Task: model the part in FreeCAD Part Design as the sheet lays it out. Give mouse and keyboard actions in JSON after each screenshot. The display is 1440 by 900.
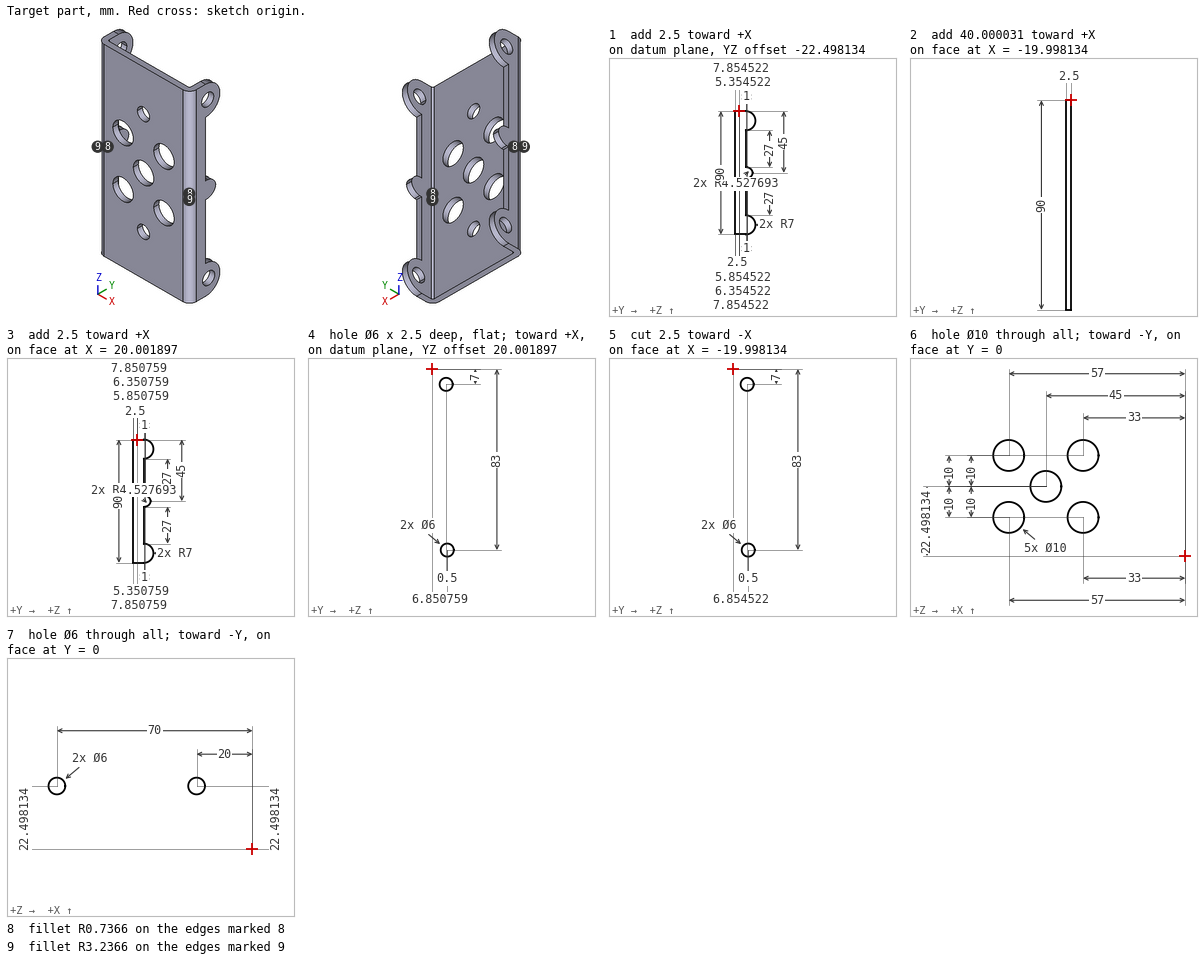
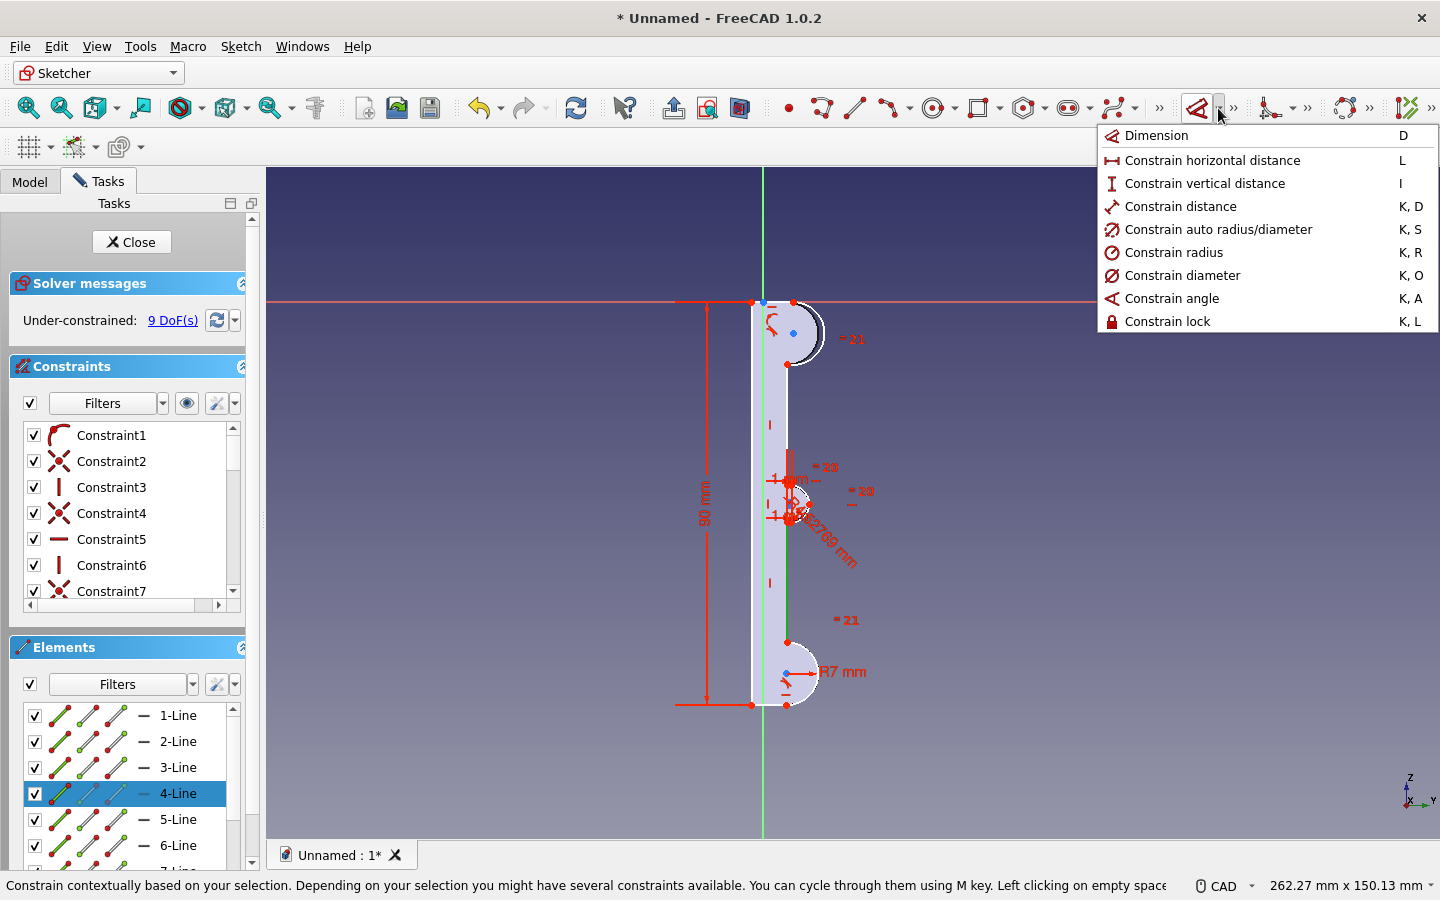
{"action": "left_click", "coordinate": [1268, 184]}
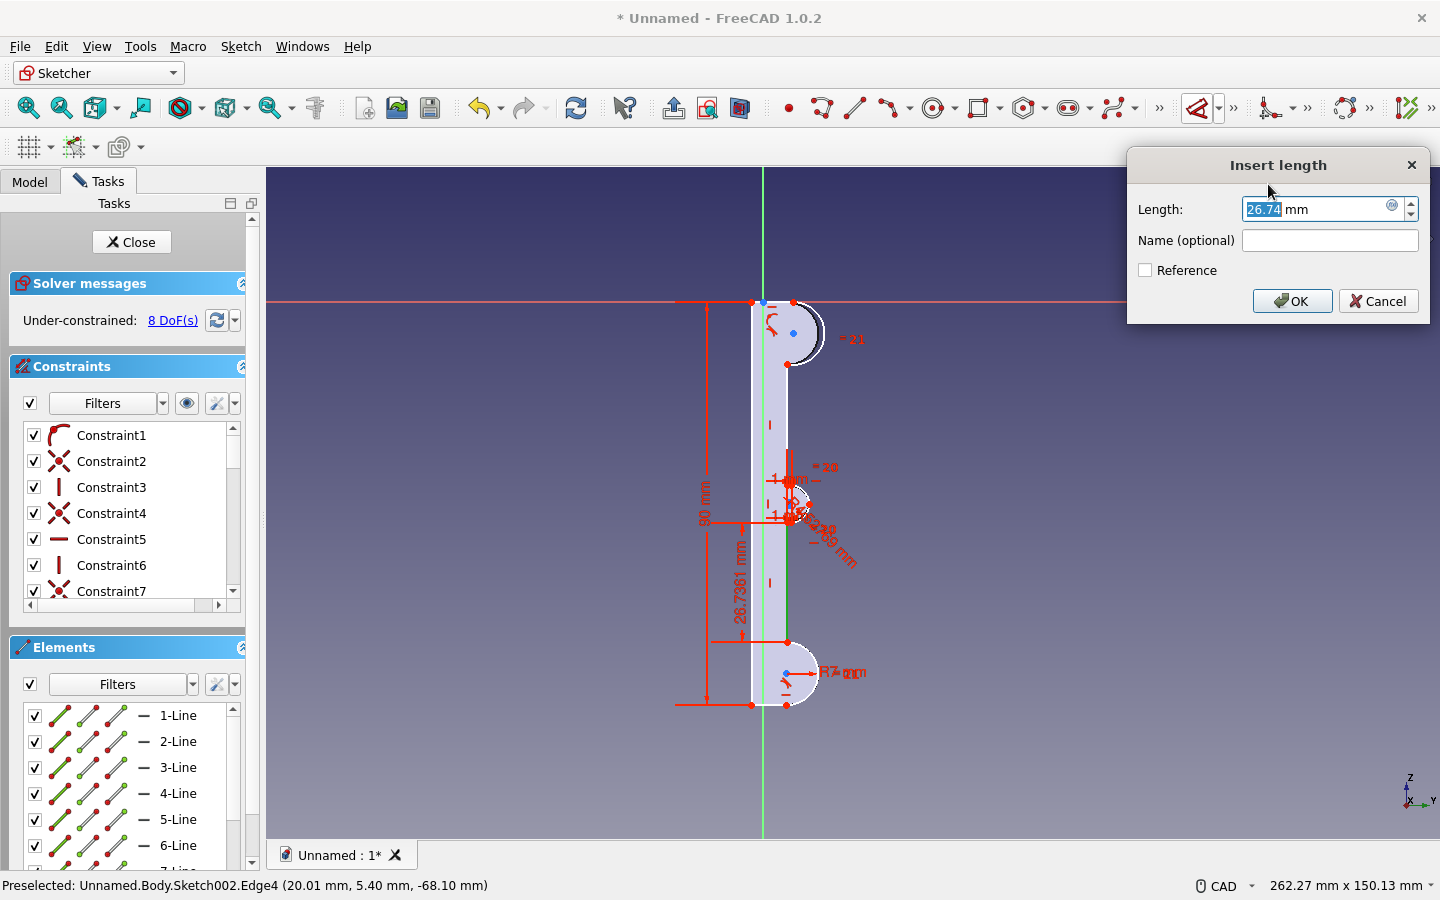
{"action": "type", "text": "27"}
{"action": "key", "text": "Return"}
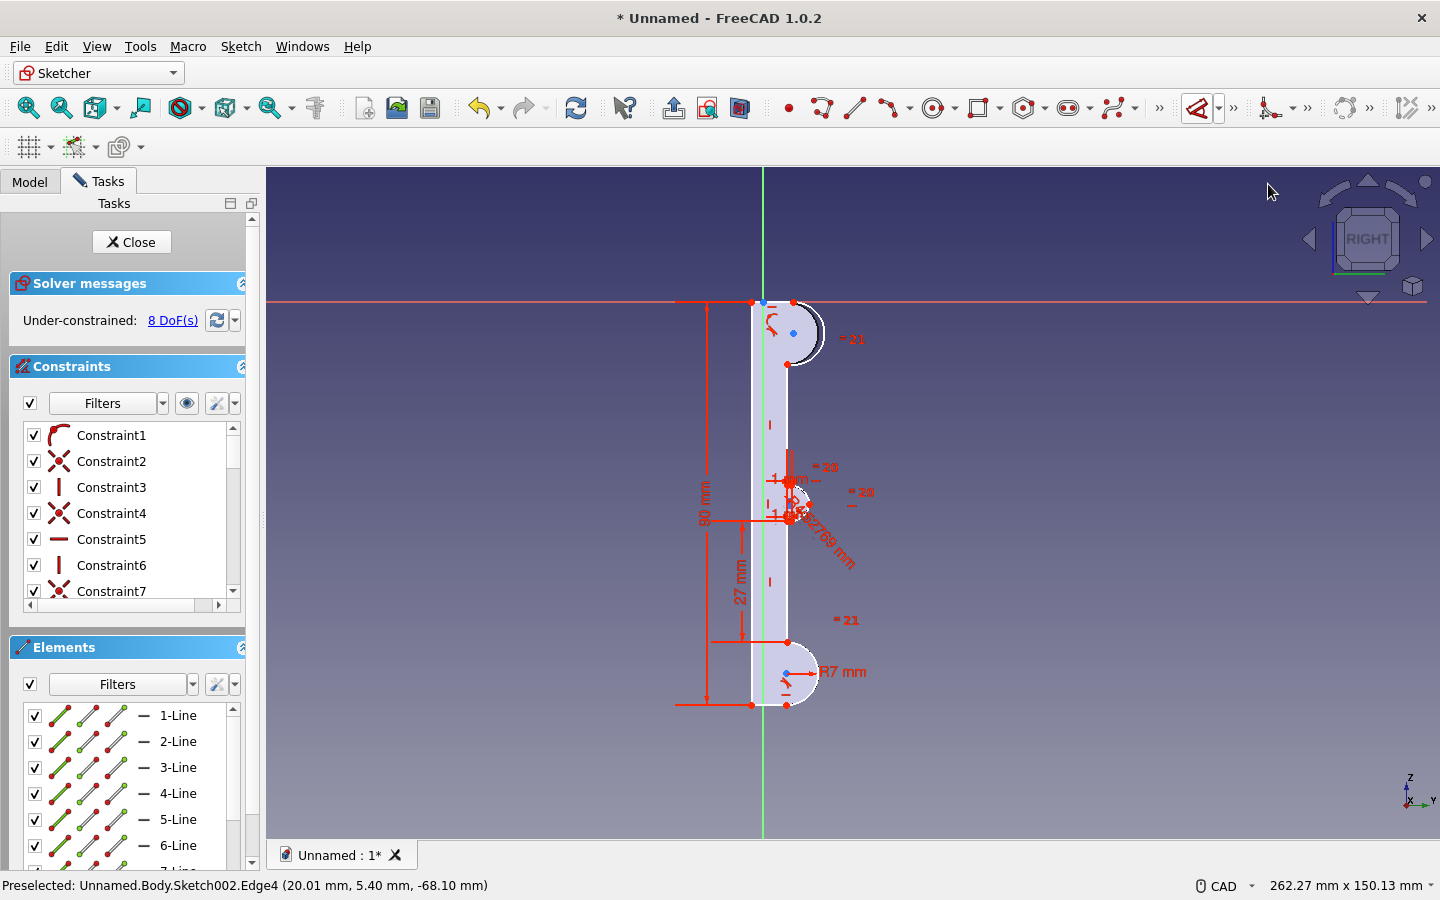
{"action": "left_click", "coordinate": [787, 449]}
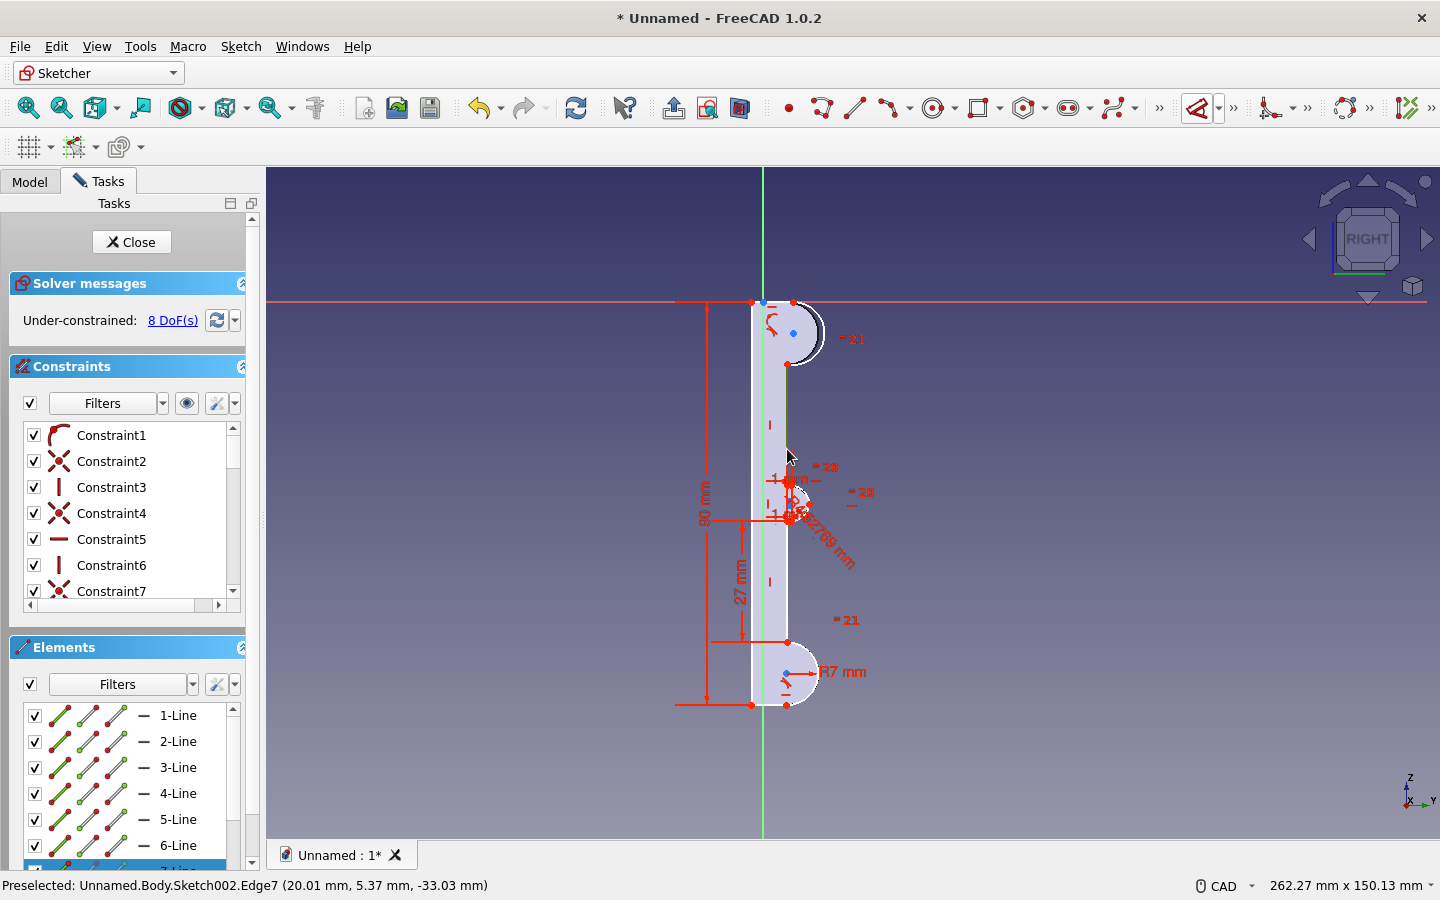
{"action": "left_click", "coordinate": [1218, 108]}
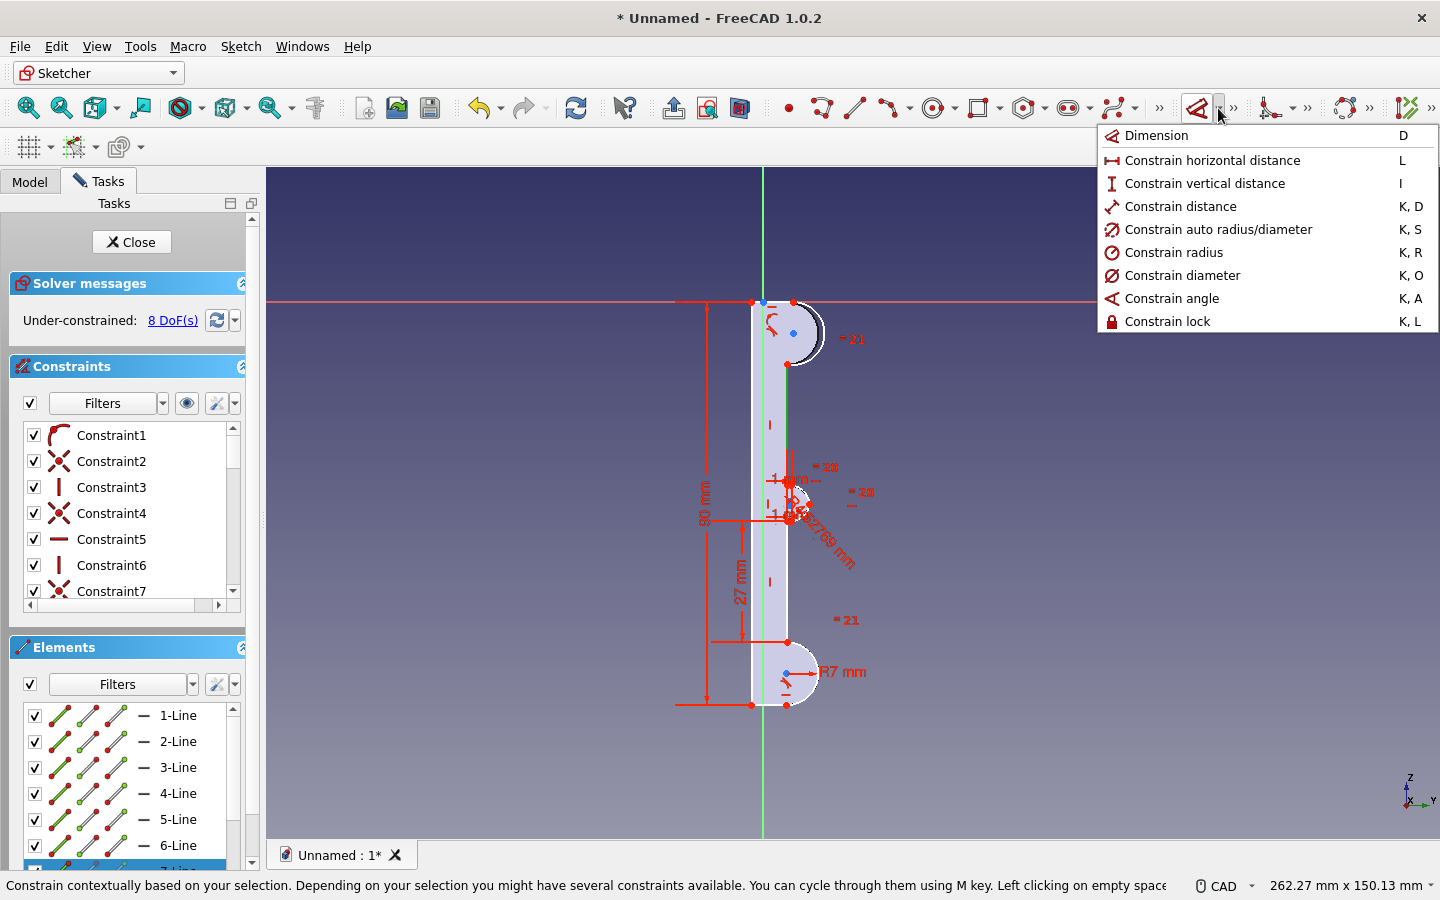
{"action": "left_click", "coordinate": [1268, 184]}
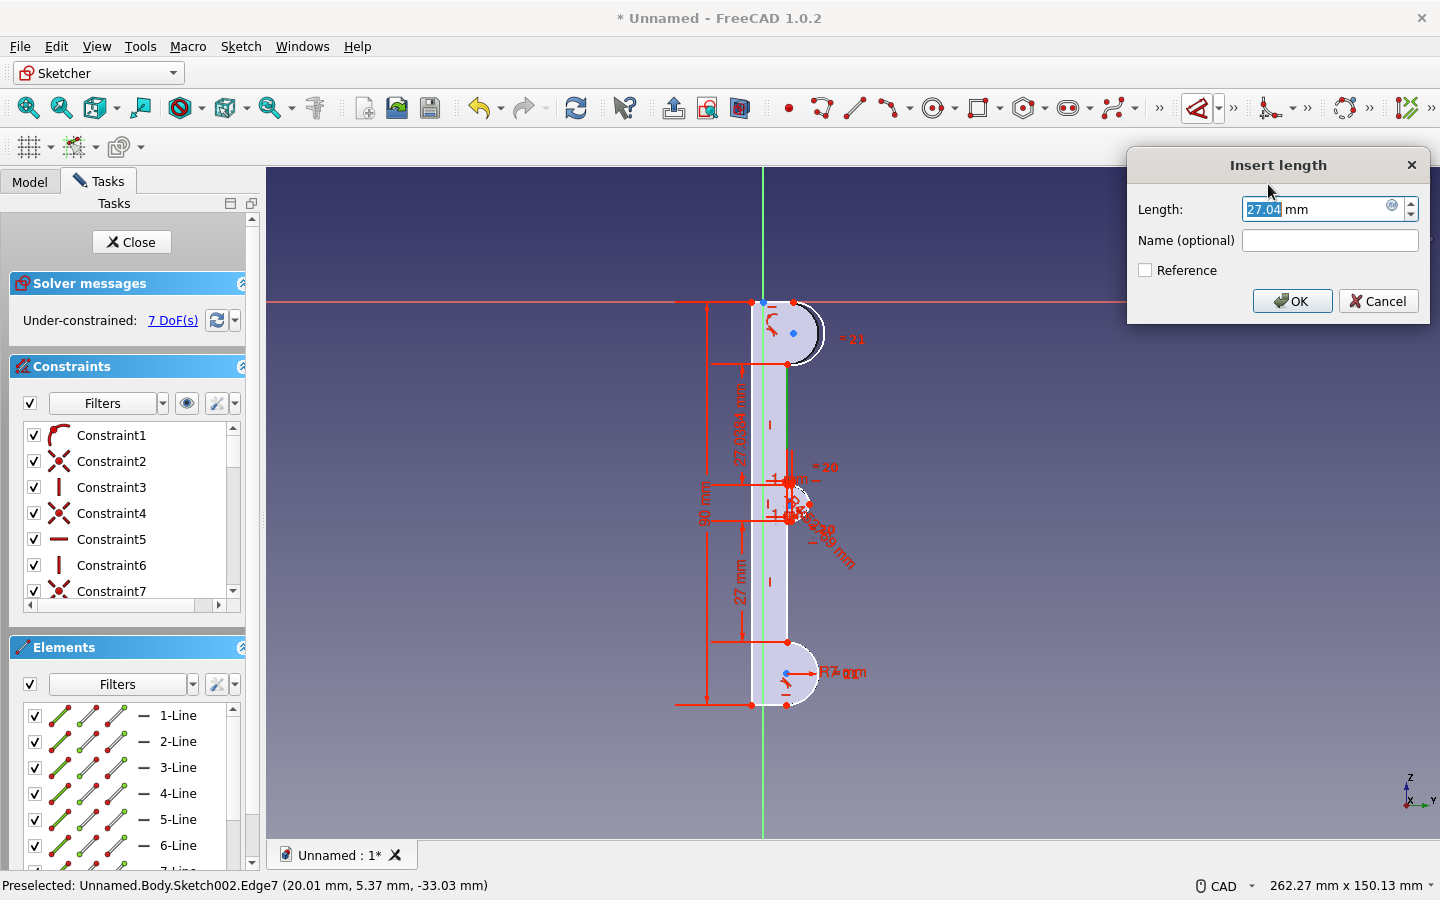
{"action": "type", "text": "27"}
{"action": "key", "text": "Return"}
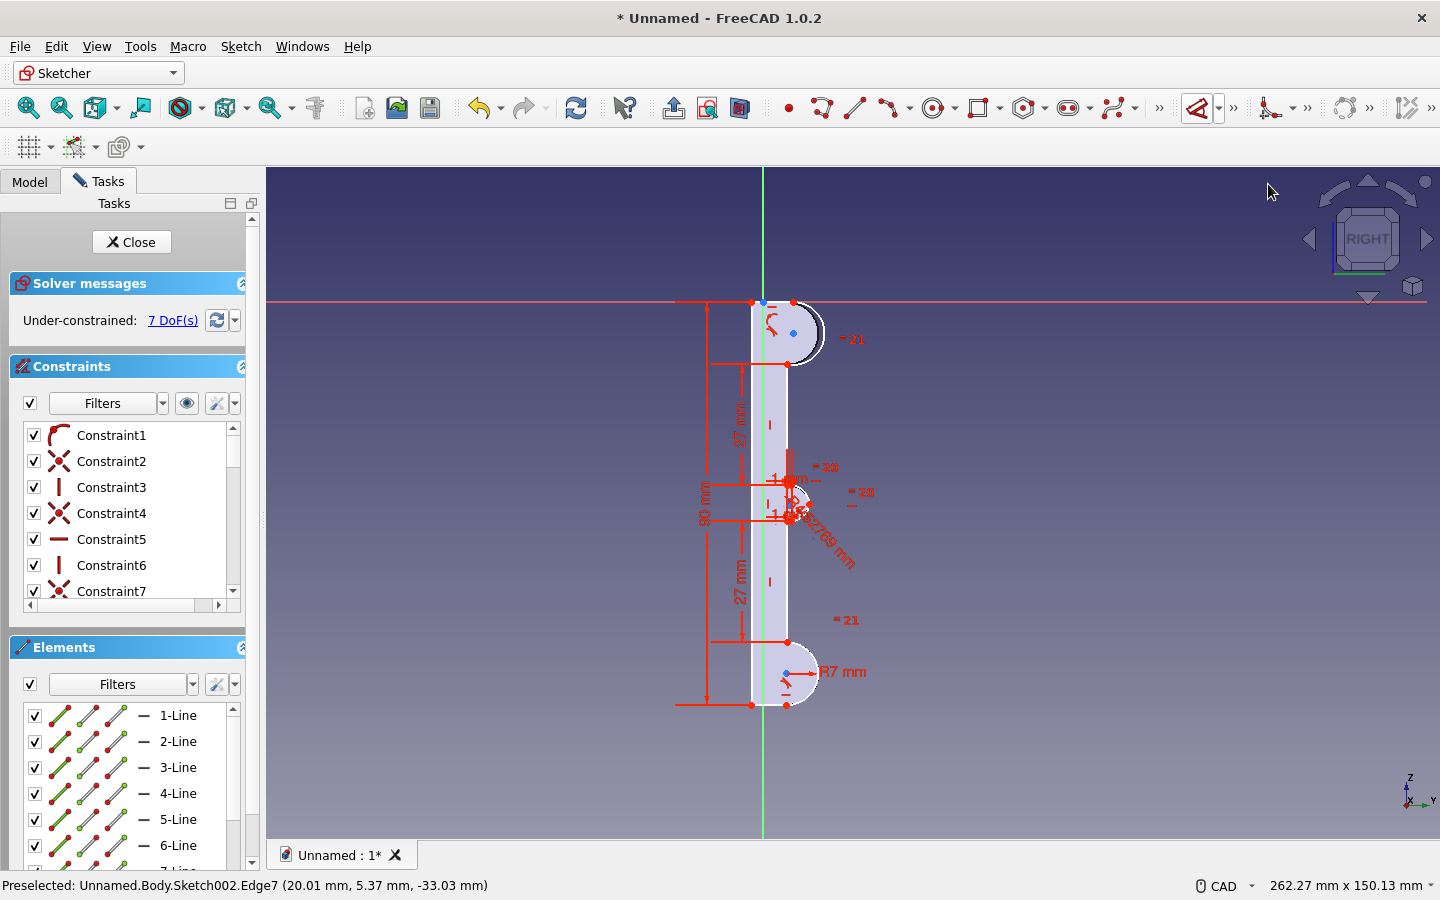
{"action": "left_click", "coordinate": [809, 505]}